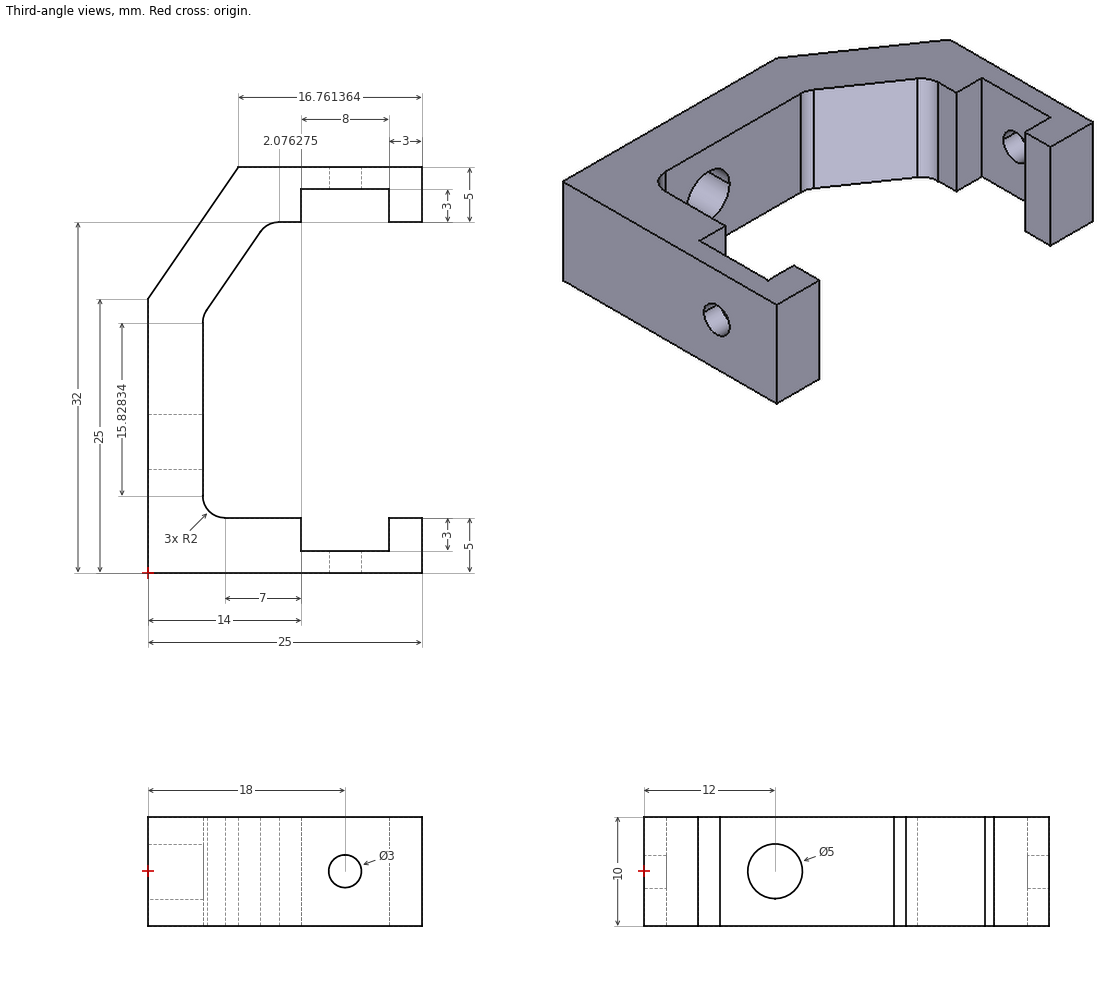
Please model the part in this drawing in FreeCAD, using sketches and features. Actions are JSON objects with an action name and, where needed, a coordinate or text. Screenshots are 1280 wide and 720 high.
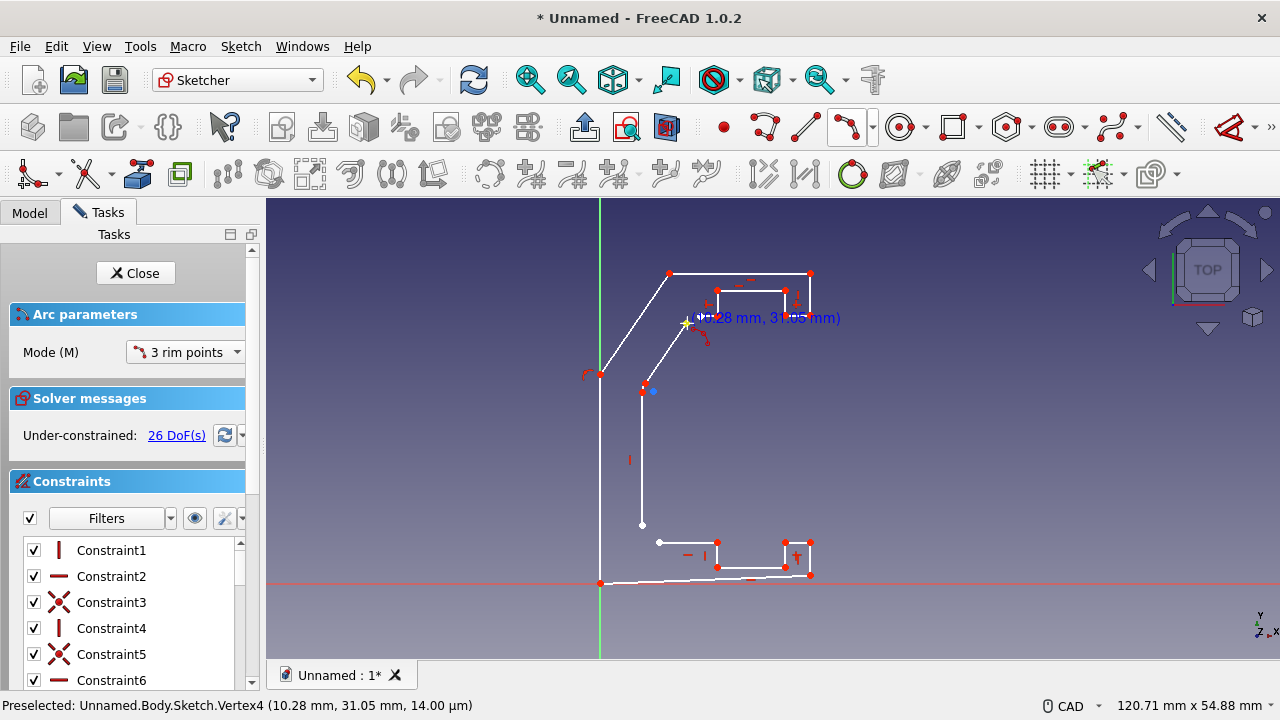
{"action": "scroll", "coordinate": [700, 315], "scroll_direction": "up", "scroll_amount": 3}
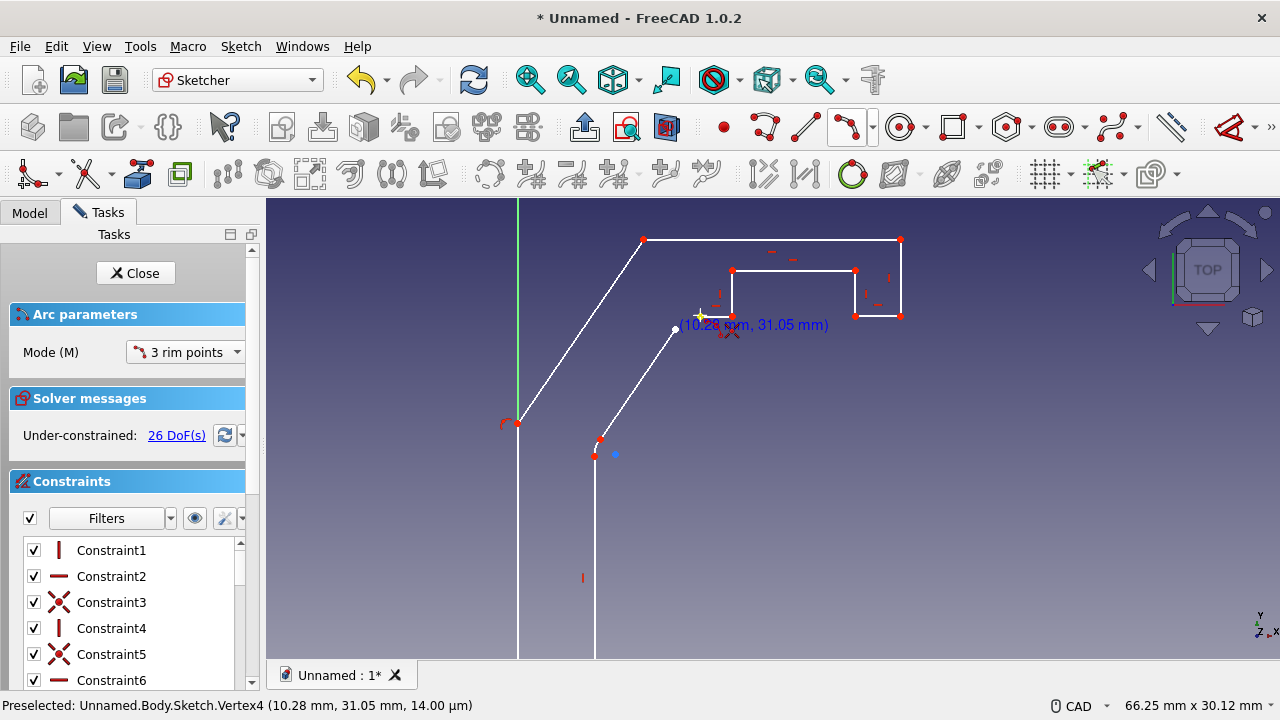
{"action": "left_click", "coordinate": [700, 317]}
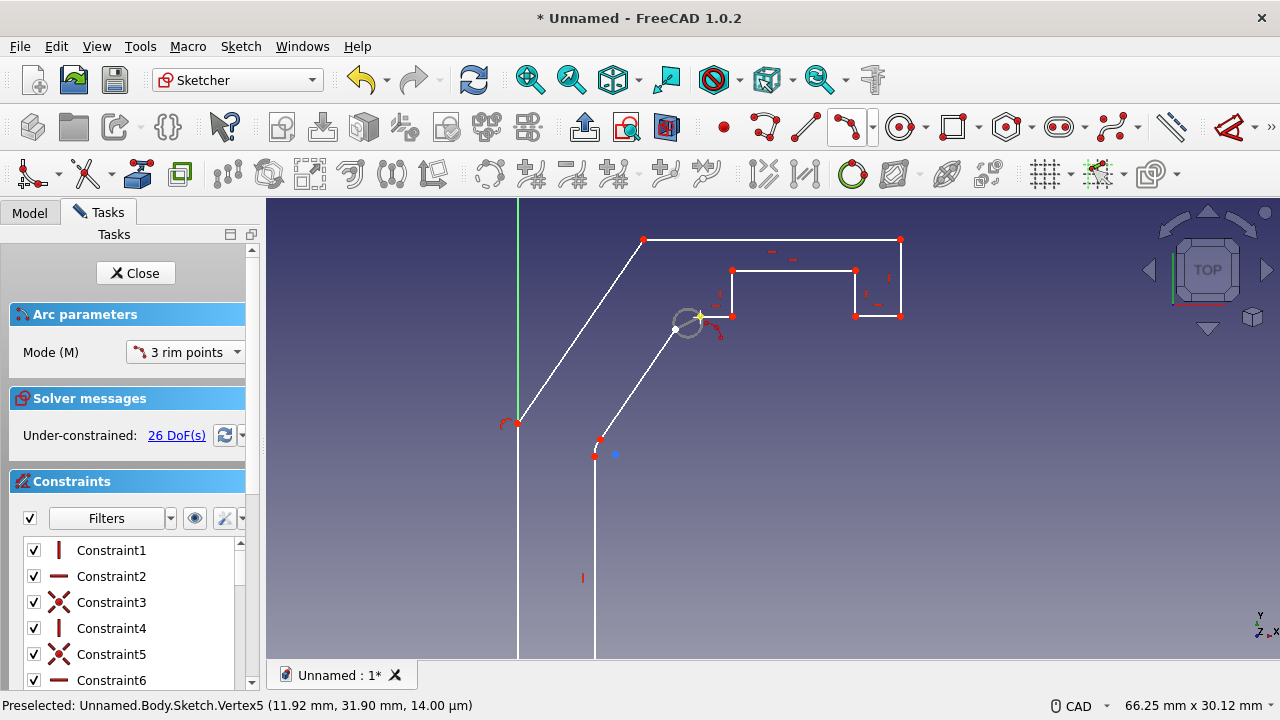
{"action": "scroll", "coordinate": [686, 319], "scroll_direction": "up", "scroll_amount": 8}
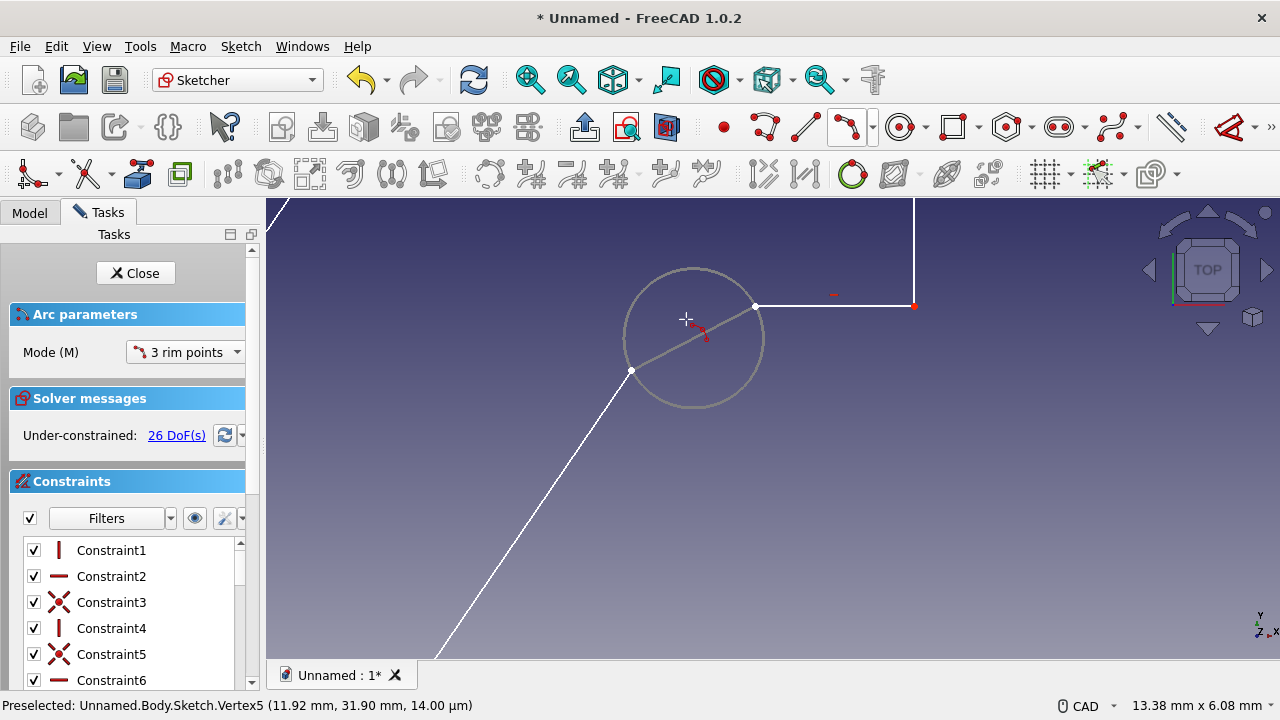
{"action": "left_click", "coordinate": [686, 316]}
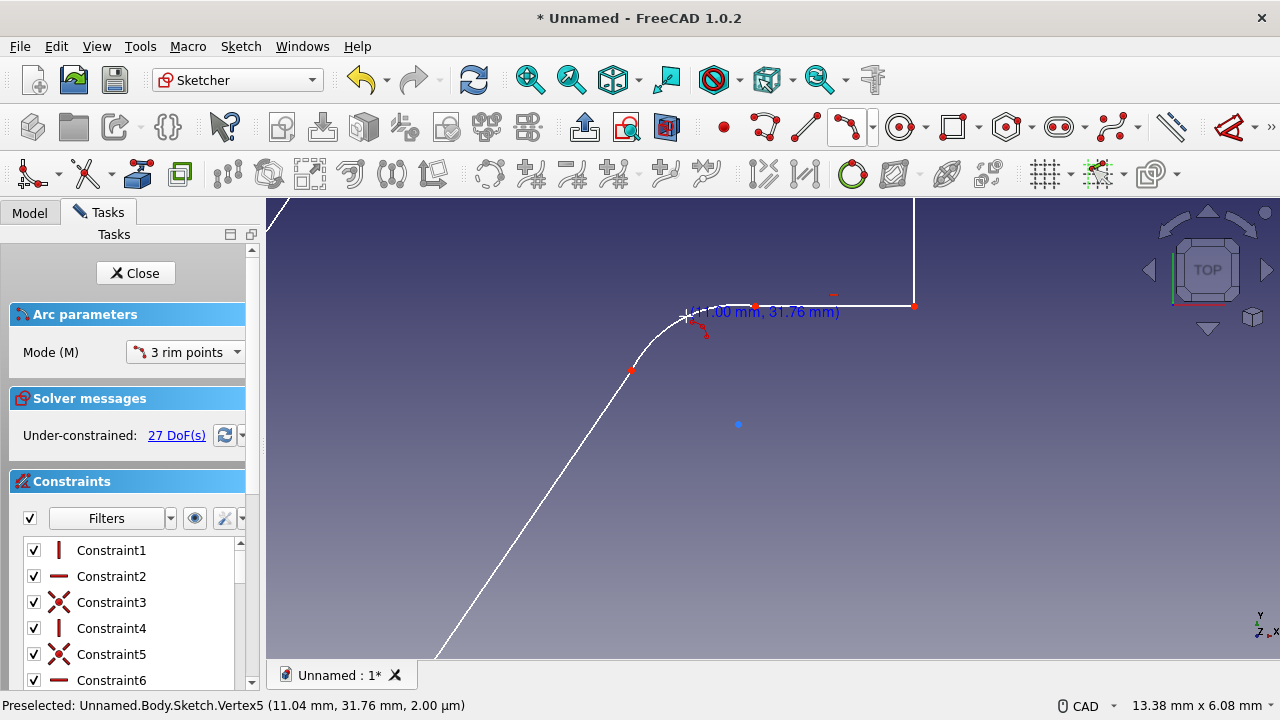
{"action": "scroll", "coordinate": [693, 317], "scroll_direction": "down", "scroll_amount": 11}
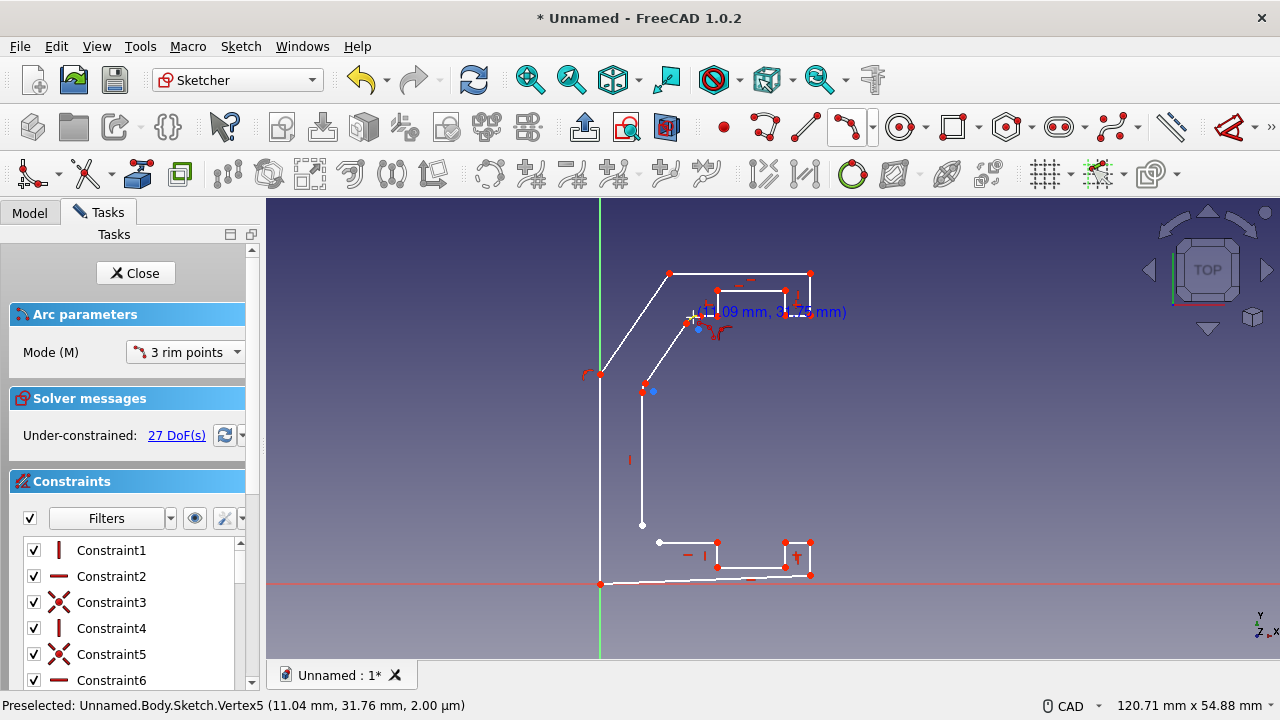
{"action": "left_click", "coordinate": [659, 543]}
{"action": "left_click", "coordinate": [642, 526]}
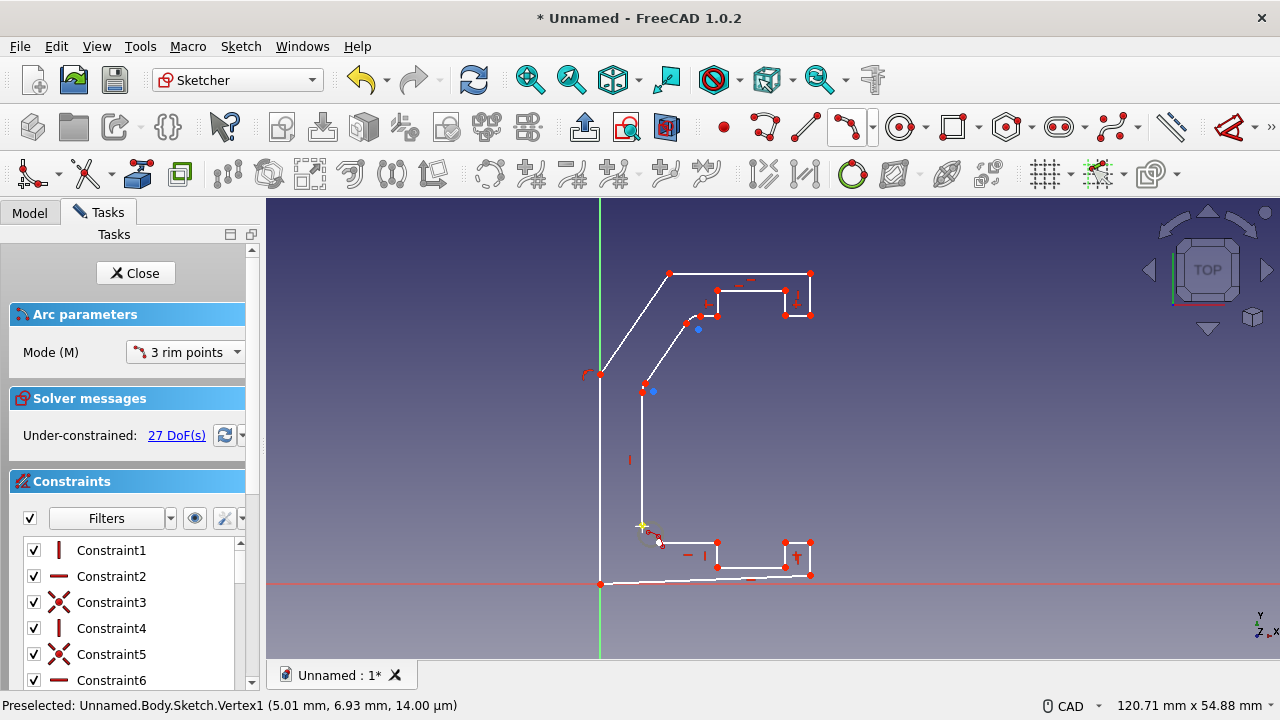
{"action": "scroll", "coordinate": [647, 537], "scroll_direction": "up", "scroll_amount": 6}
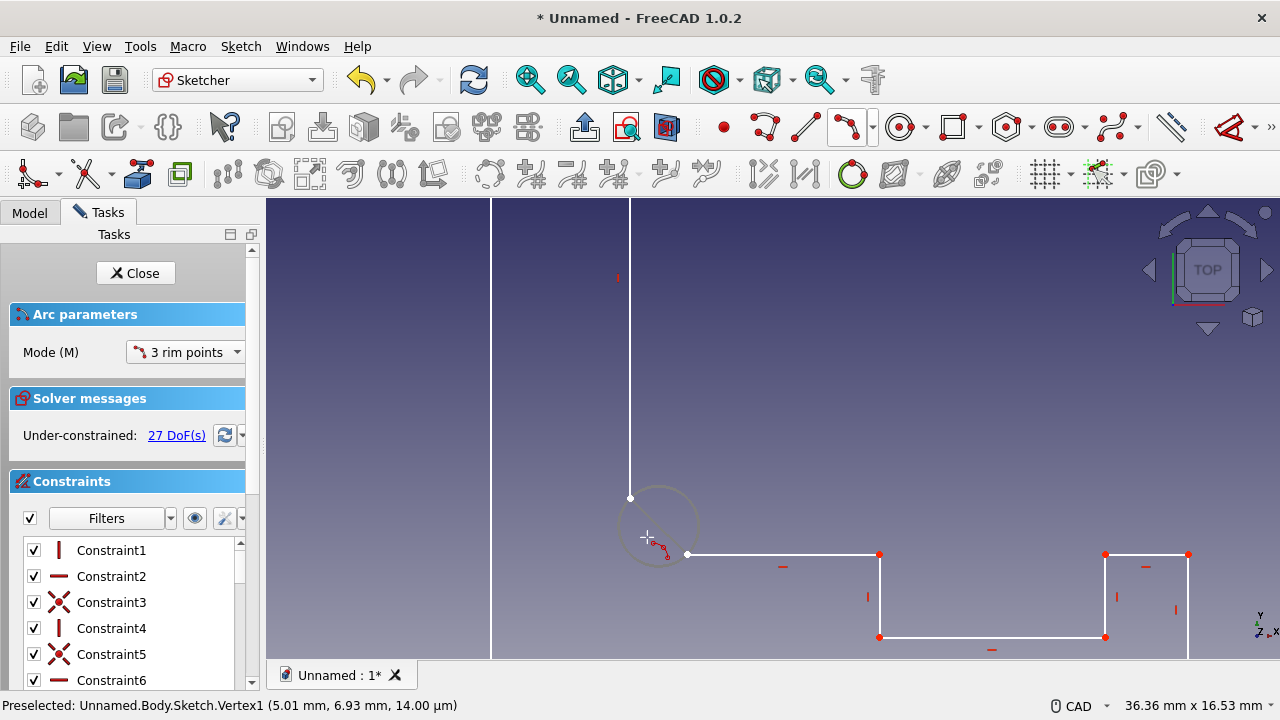
{"action": "left_click", "coordinate": [647, 536]}
{"action": "key", "text": "Escape"}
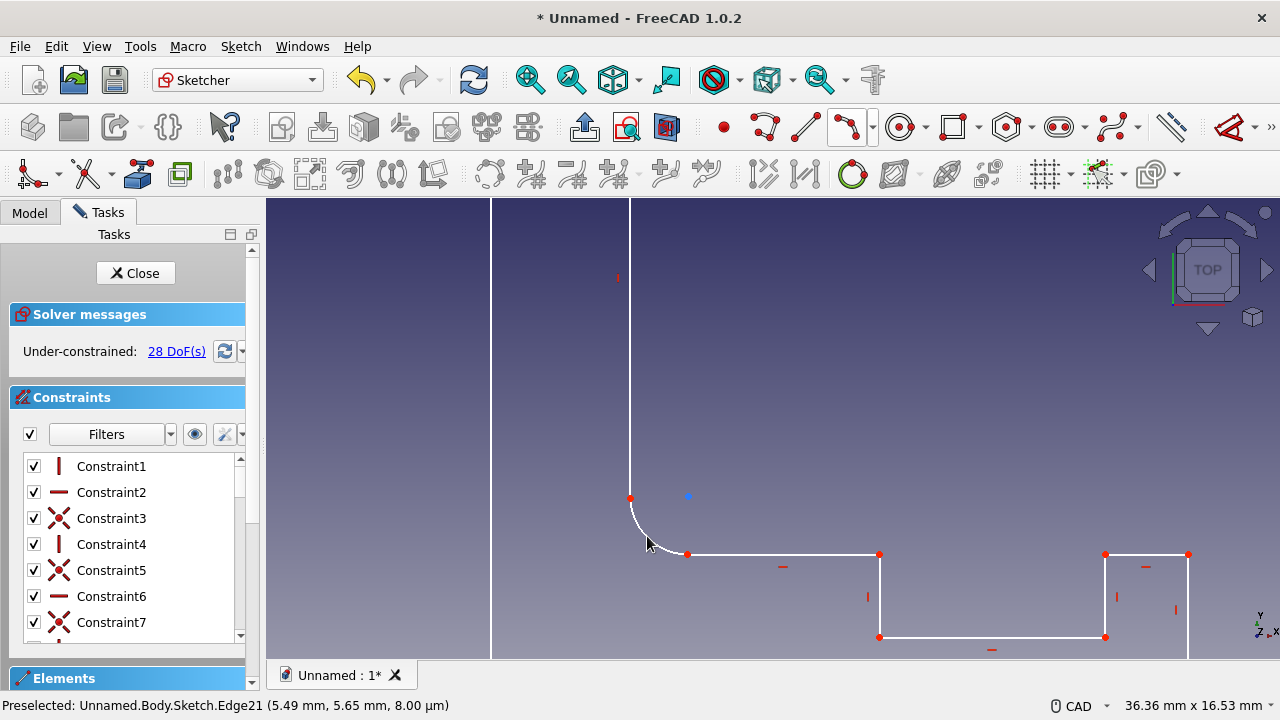
{"action": "left_click", "coordinate": [630, 366]}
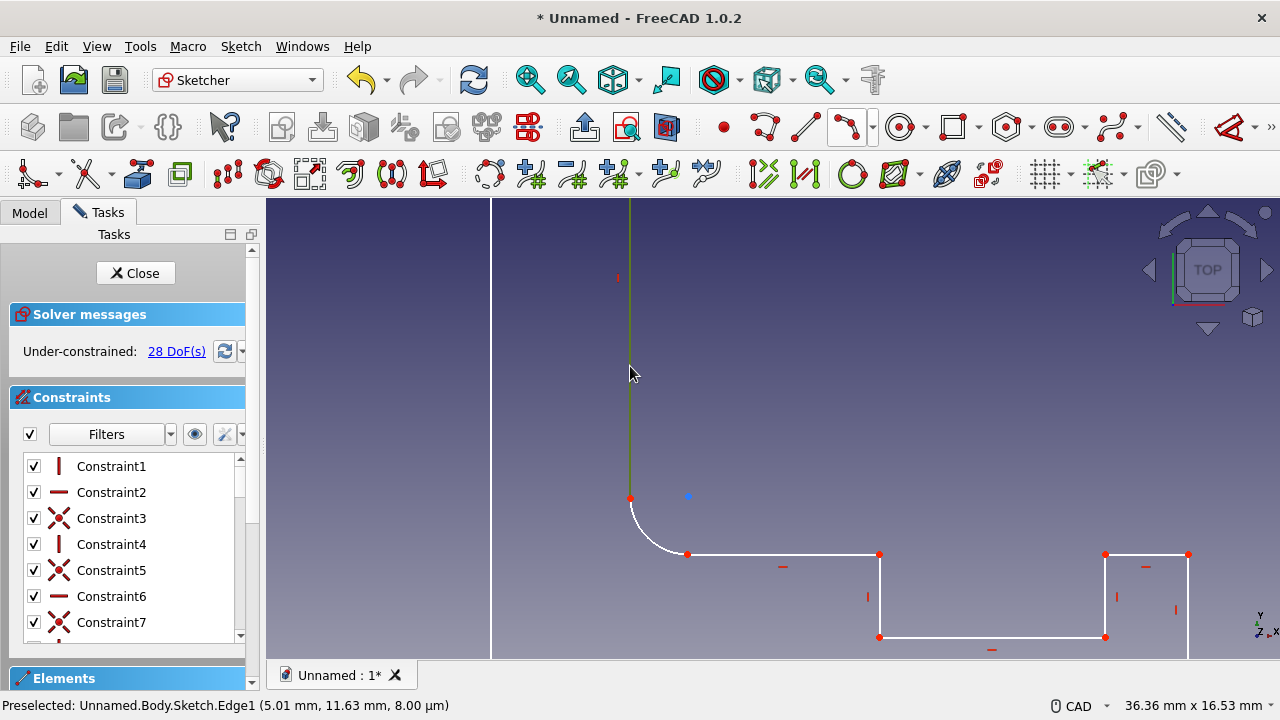
{"action": "scroll", "coordinate": [646, 538], "scroll_direction": "down", "scroll_amount": 6}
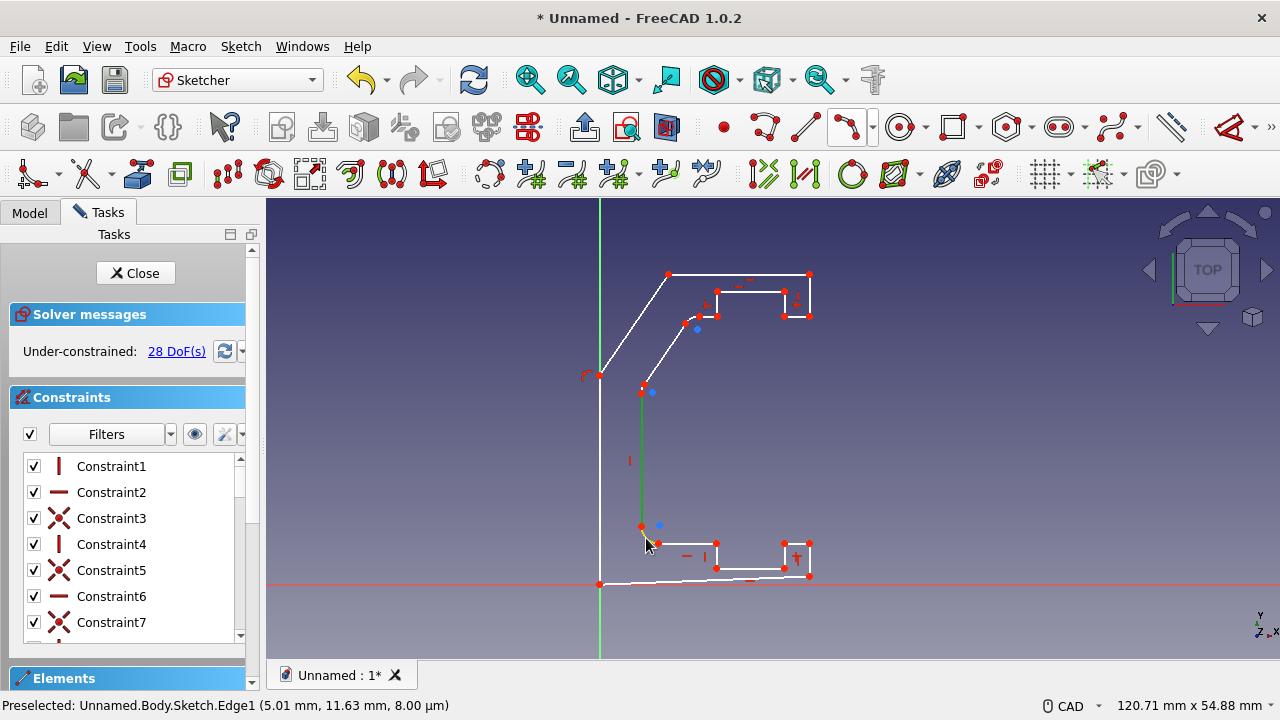
{"action": "scroll", "coordinate": [643, 387], "scroll_direction": "up", "scroll_amount": 8}